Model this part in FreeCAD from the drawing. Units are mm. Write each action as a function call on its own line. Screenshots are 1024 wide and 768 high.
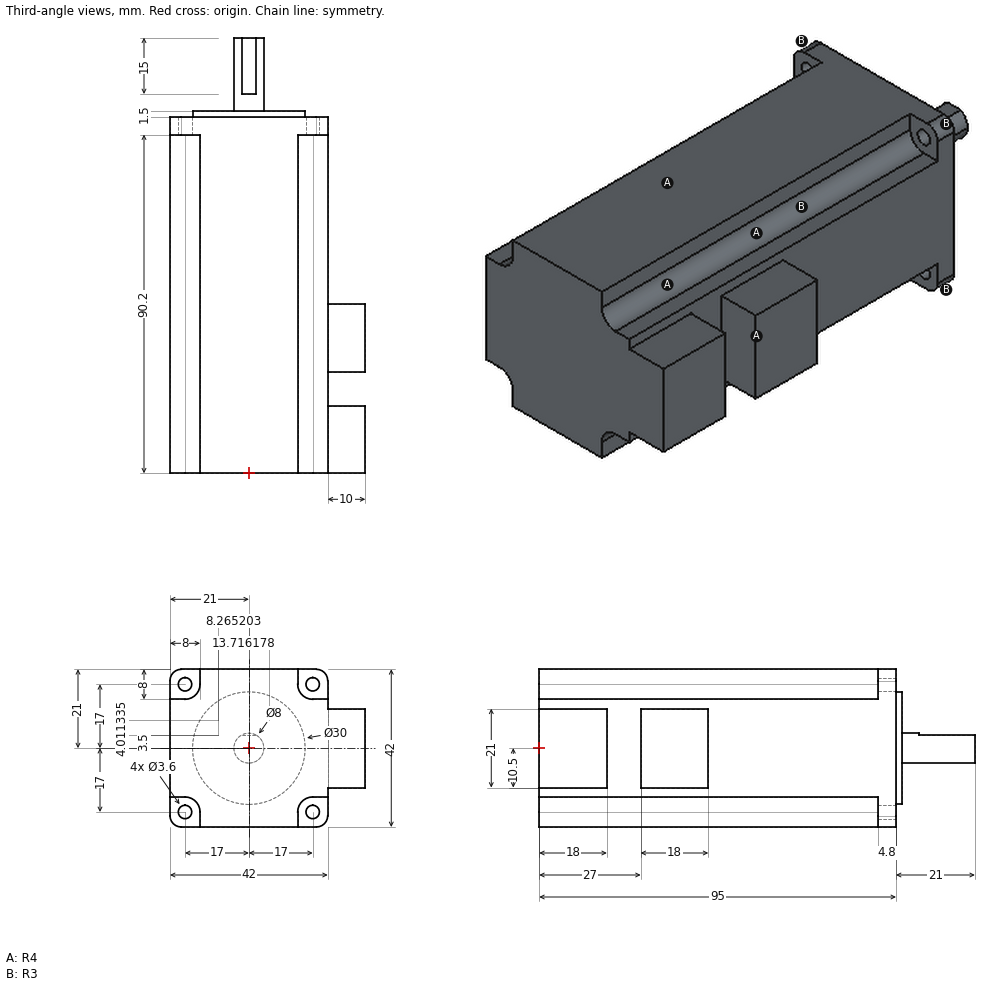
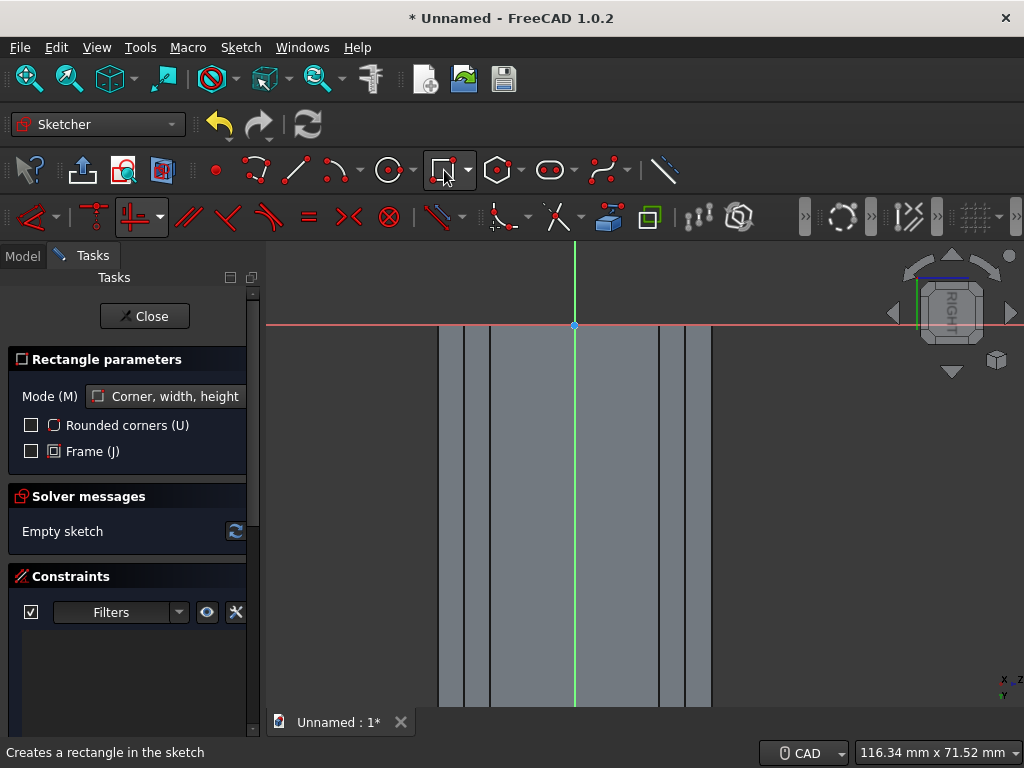
click(506, 325)
click(643, 443)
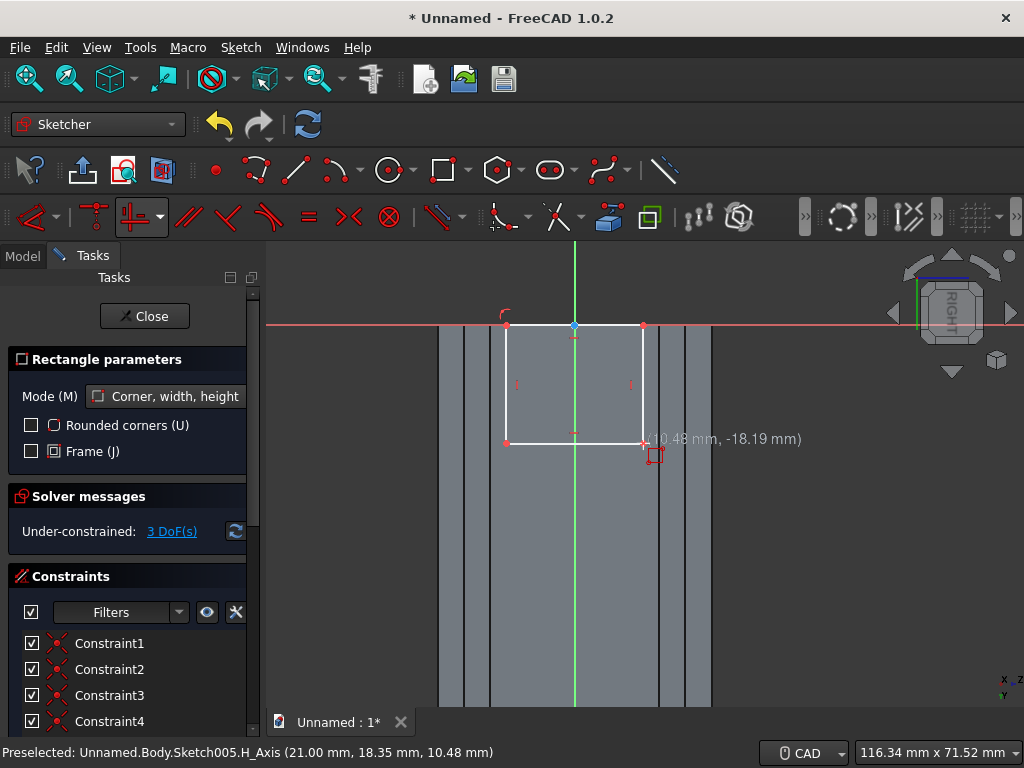
click(506, 501)
click(643, 619)
key(Escape)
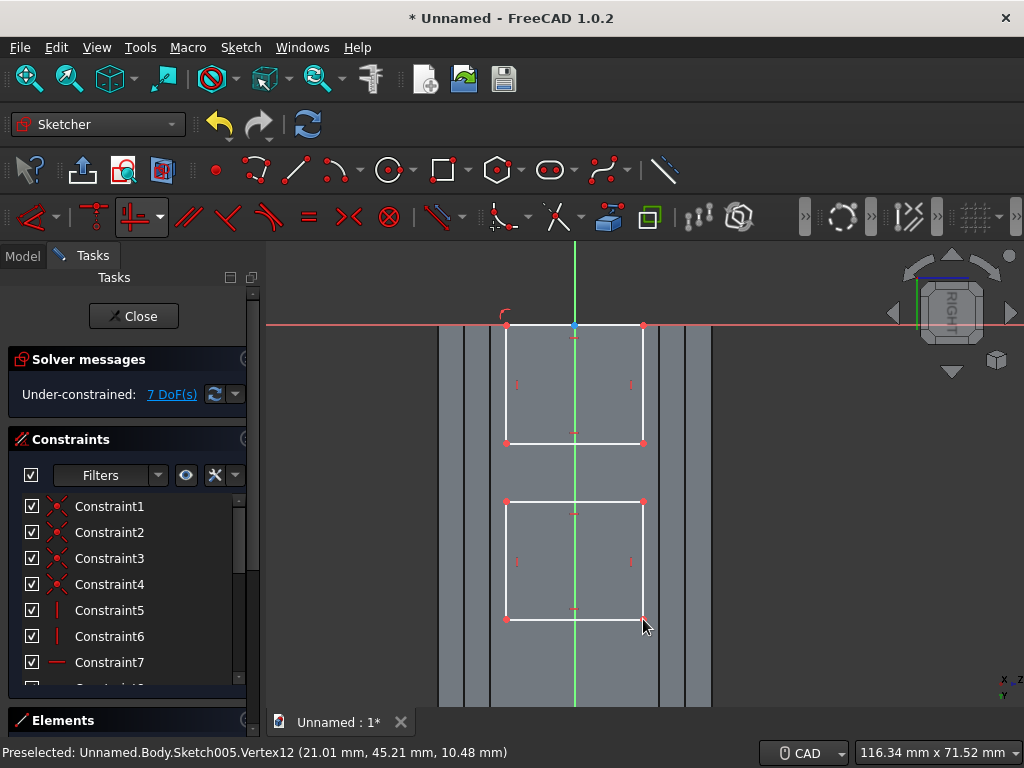
key(d)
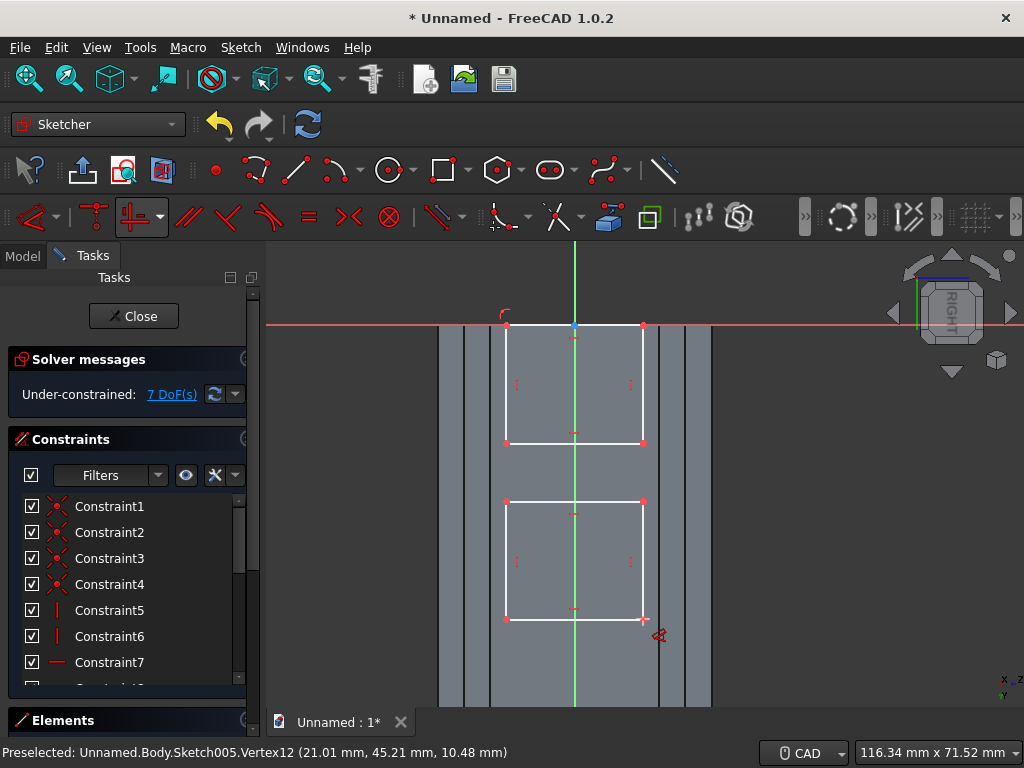
click(506, 361)
click(472, 385)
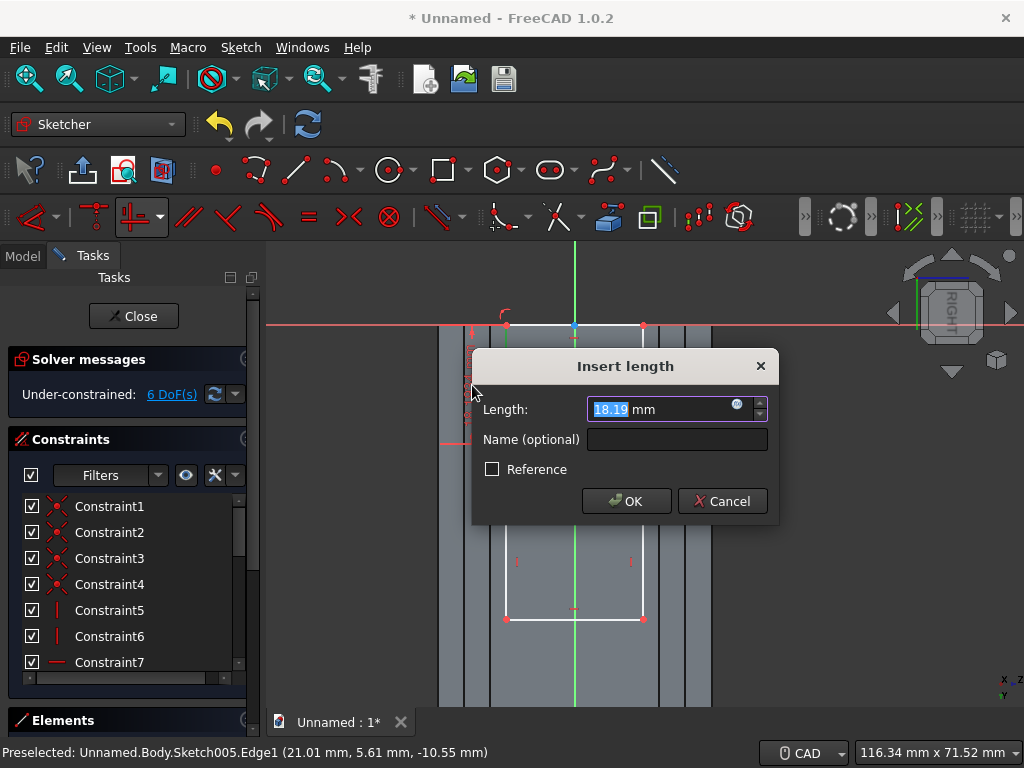
text(18)
key(Return)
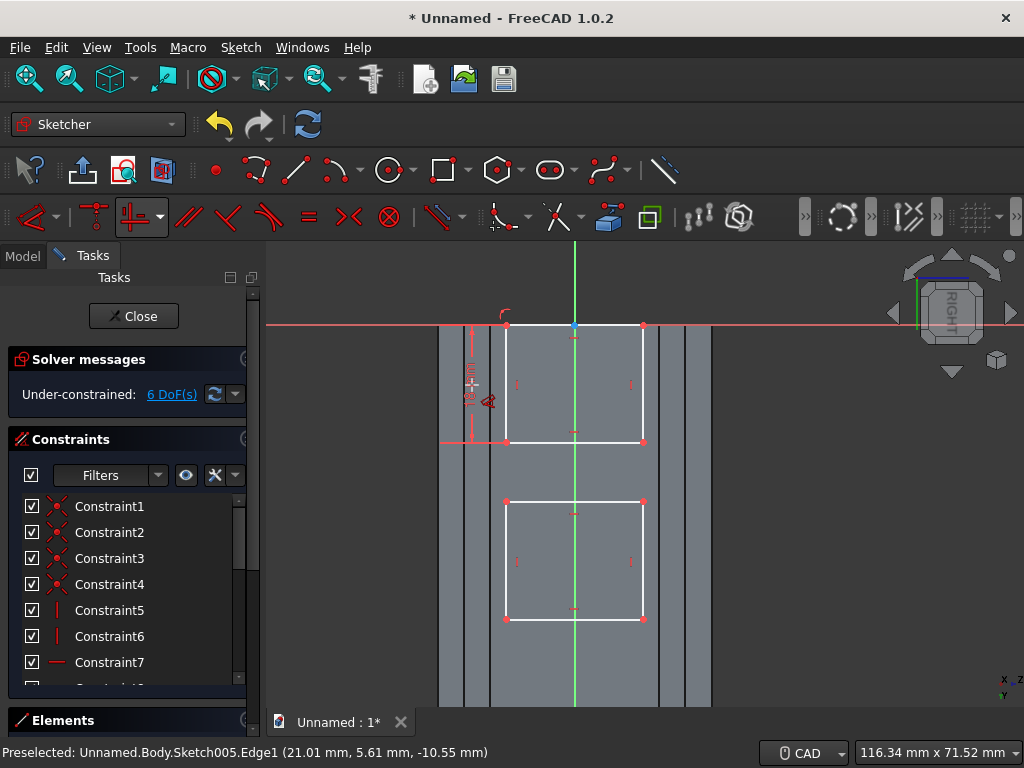
click(547, 443)
click(543, 409)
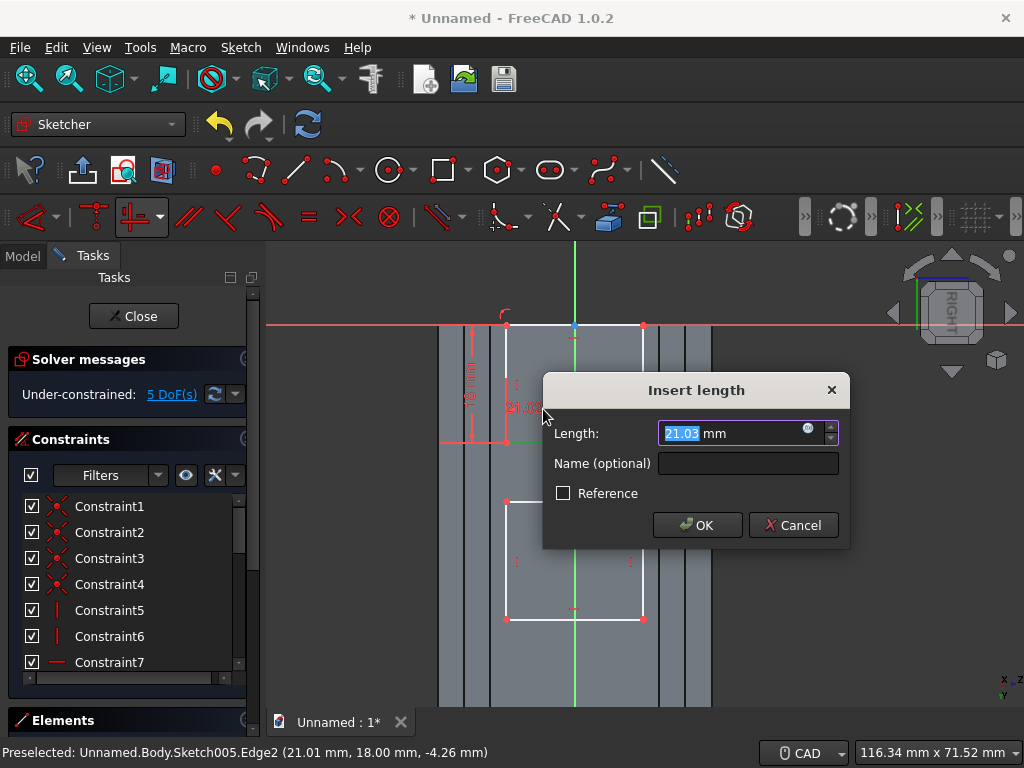
text(21)
key(Return)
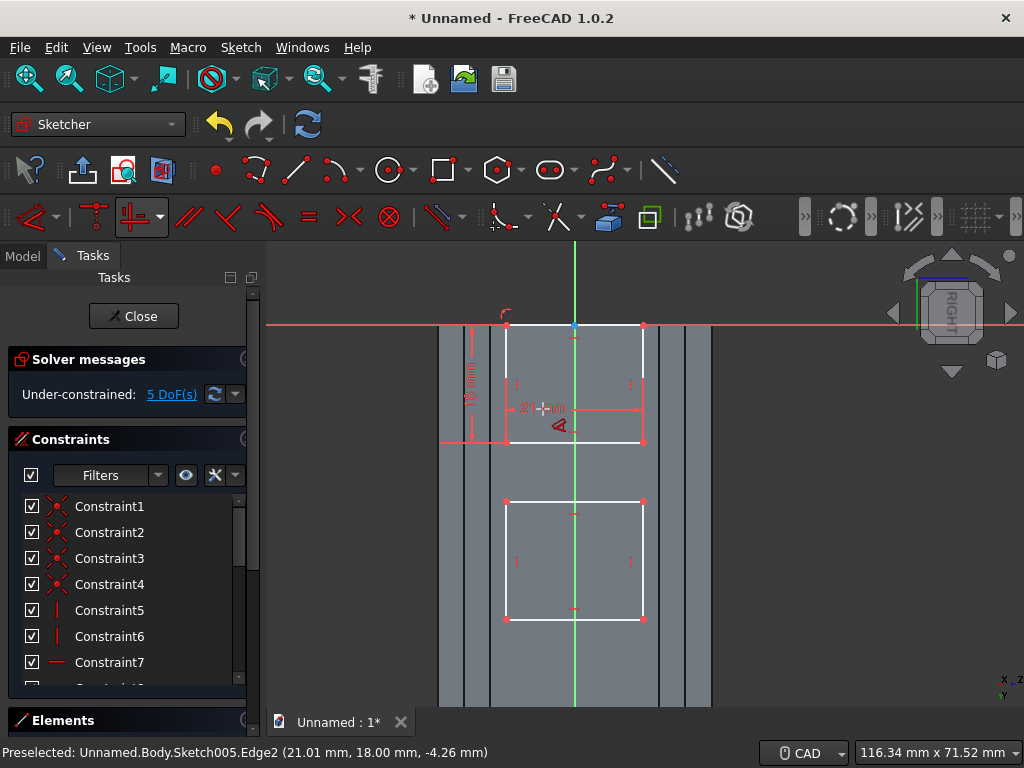
click(506, 537)
click(472, 561)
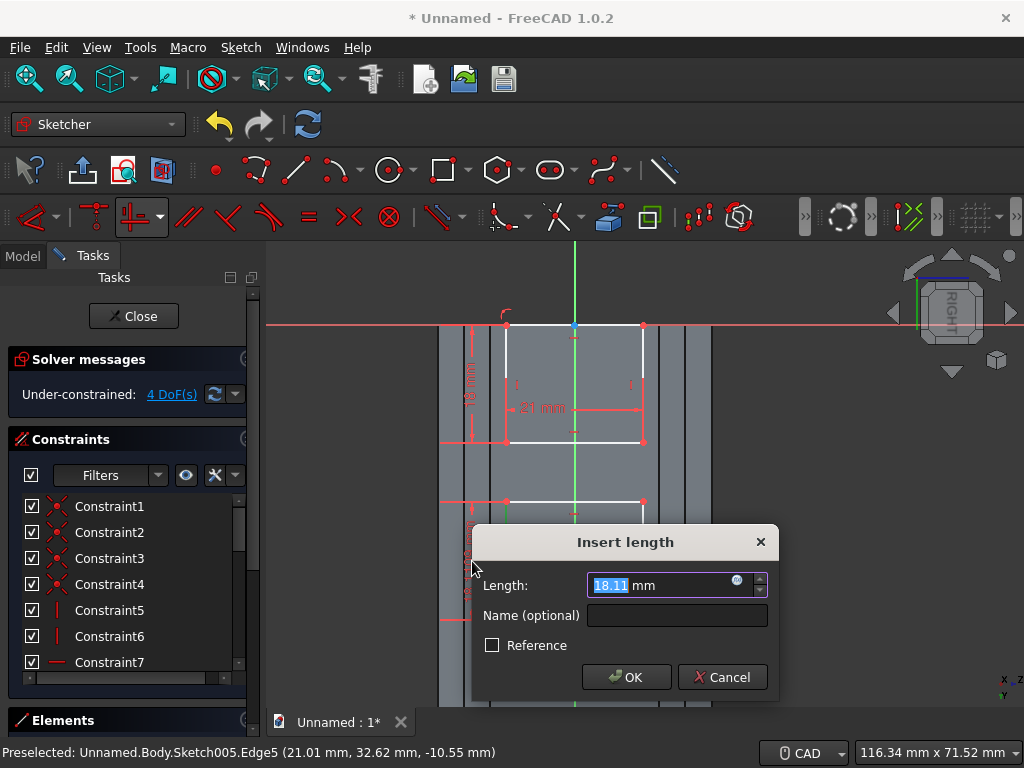
text(18)
key(Return)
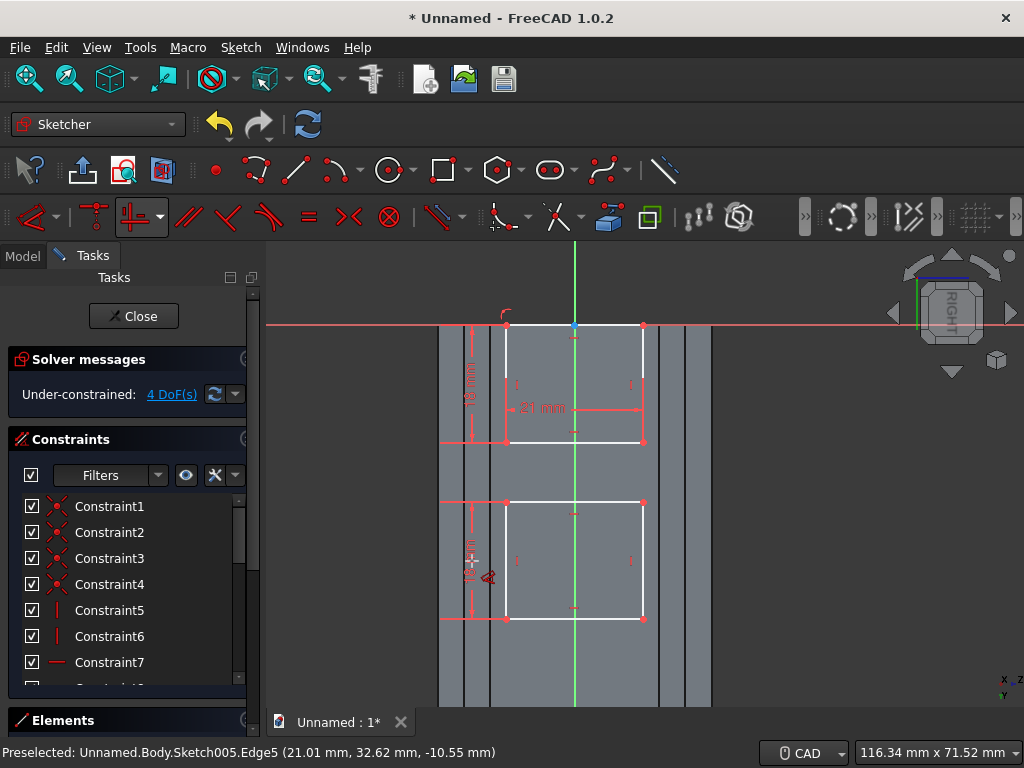
click(547, 619)
click(543, 653)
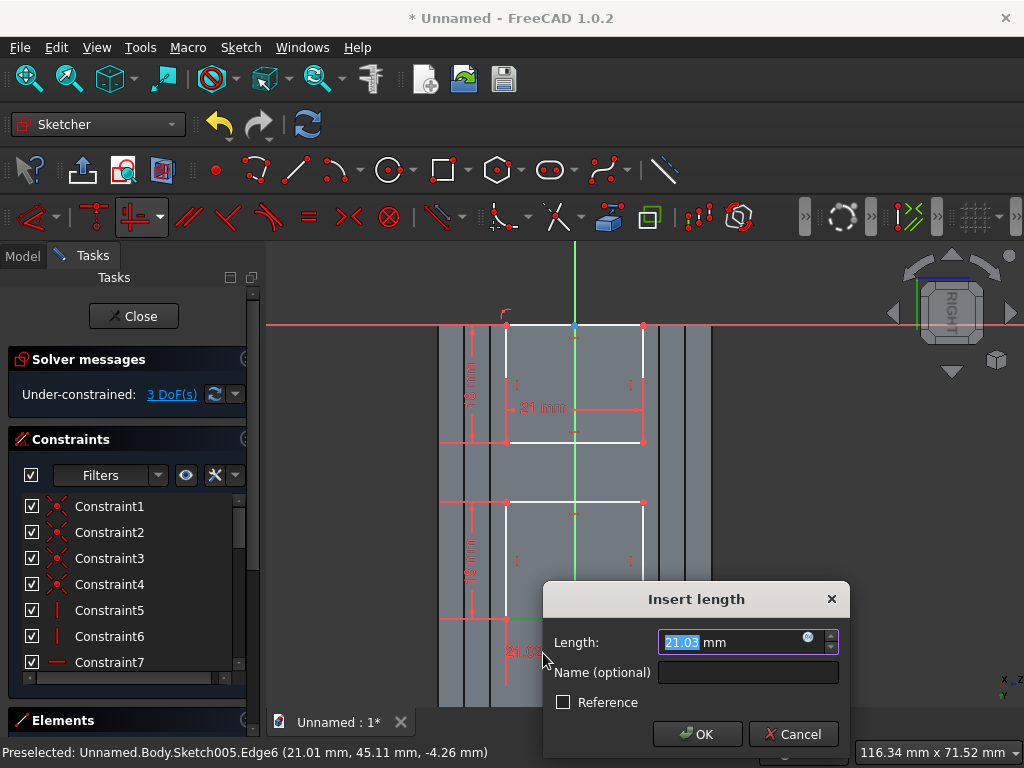
text(21)
key(Return)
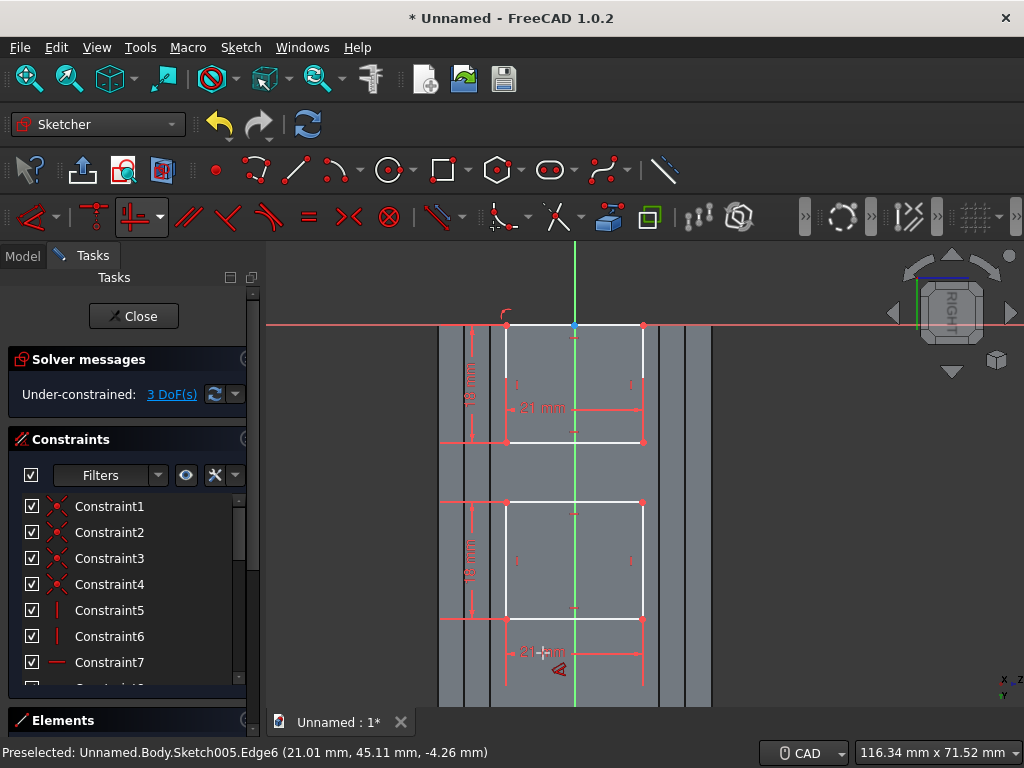
click(506, 502)
click(472, 414)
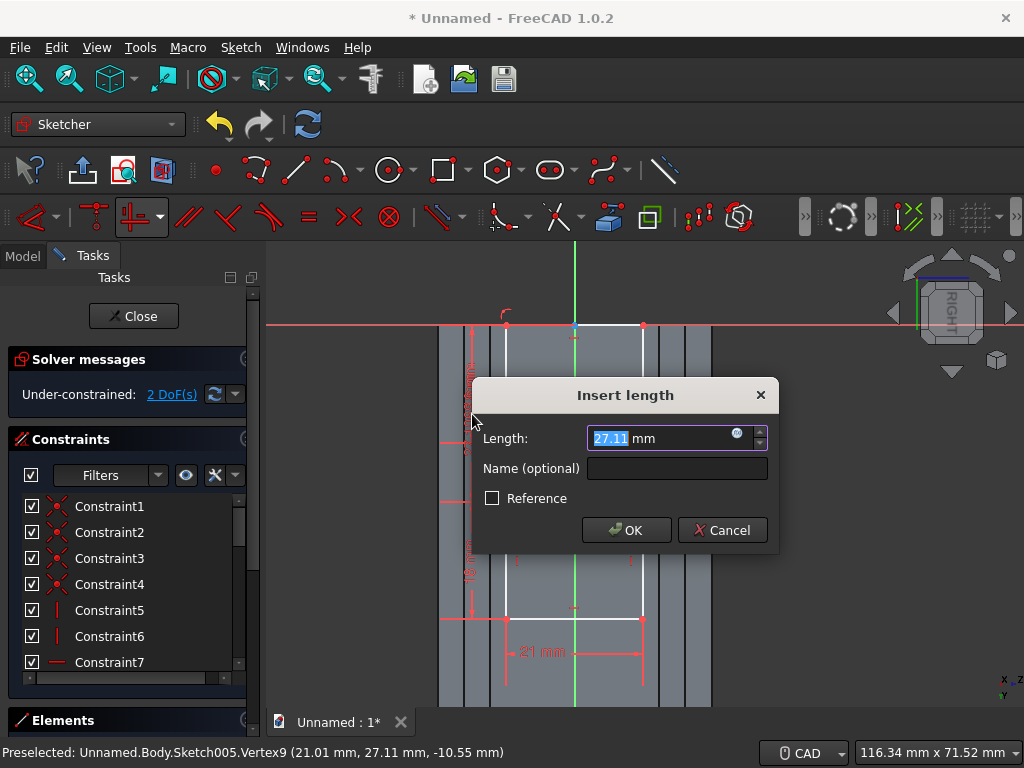
text(27)
key(Return)